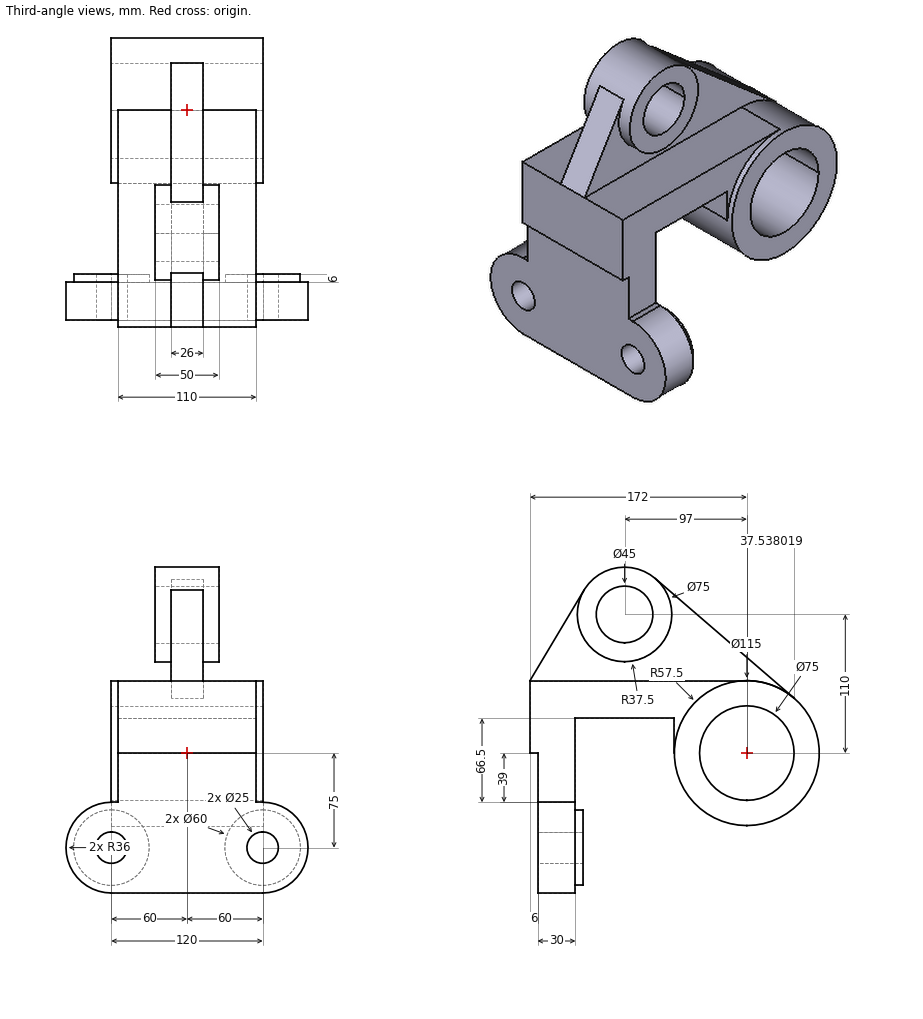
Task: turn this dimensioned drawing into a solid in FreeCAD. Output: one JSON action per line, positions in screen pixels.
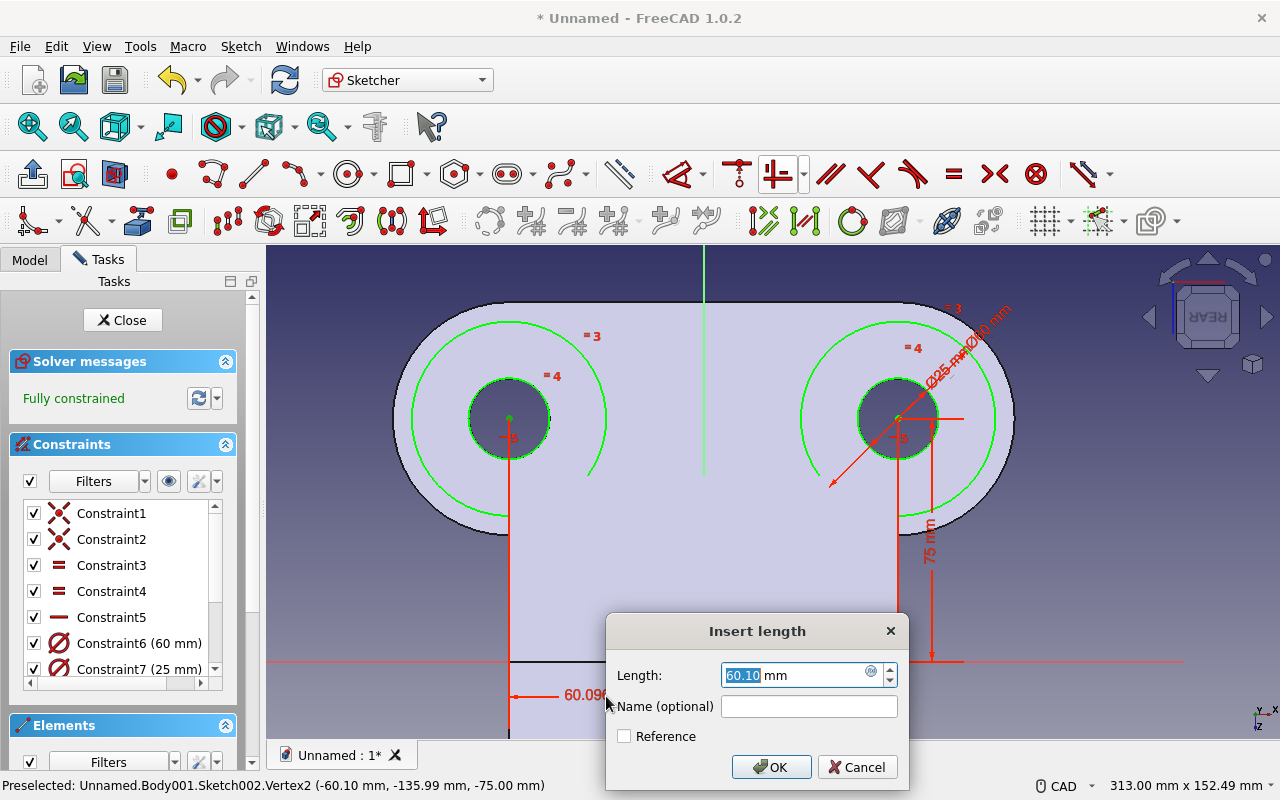
{"action": "type", "text": "60"}
{"action": "key", "text": "Return"}
{"action": "key", "text": "Escape"}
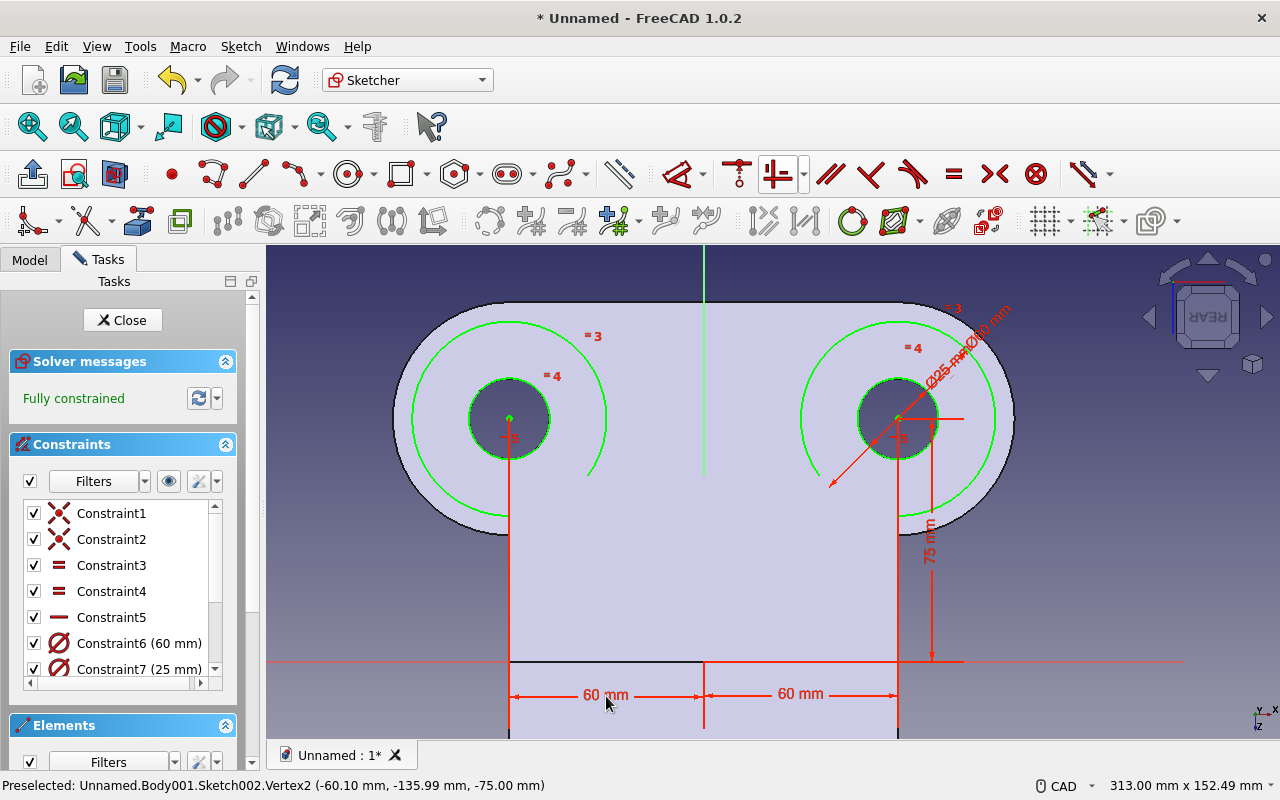
{"action": "left_click", "coordinate": [123, 320]}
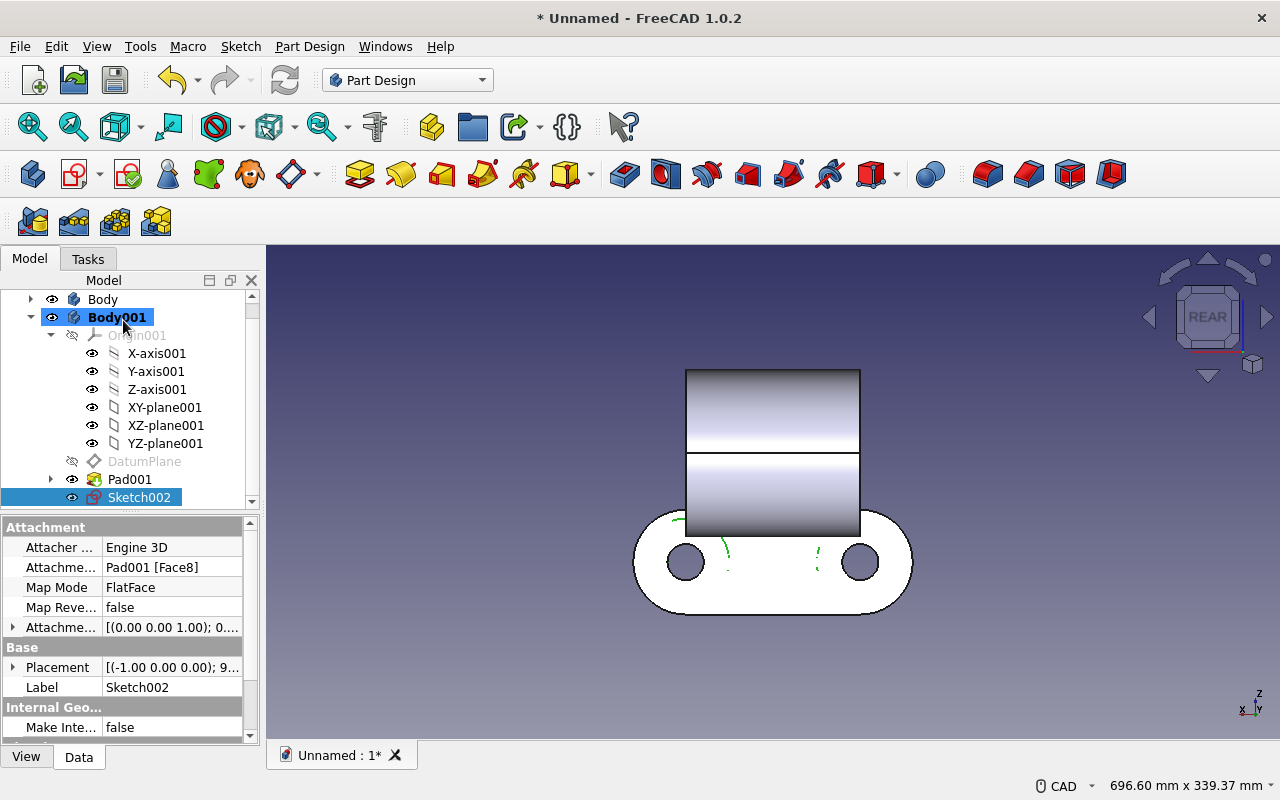
{"action": "left_click", "coordinate": [360, 174]}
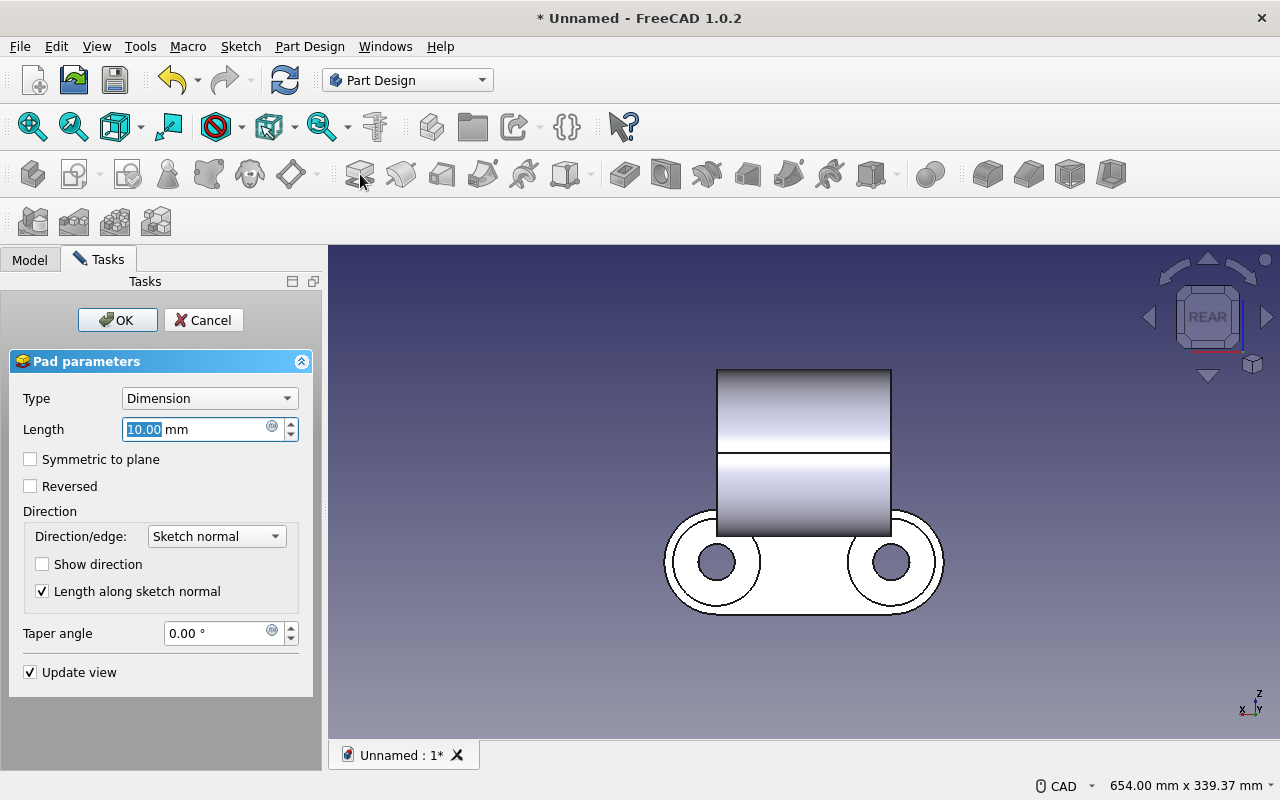
{"action": "type", "text": "6"}
{"action": "key", "text": "Tab"}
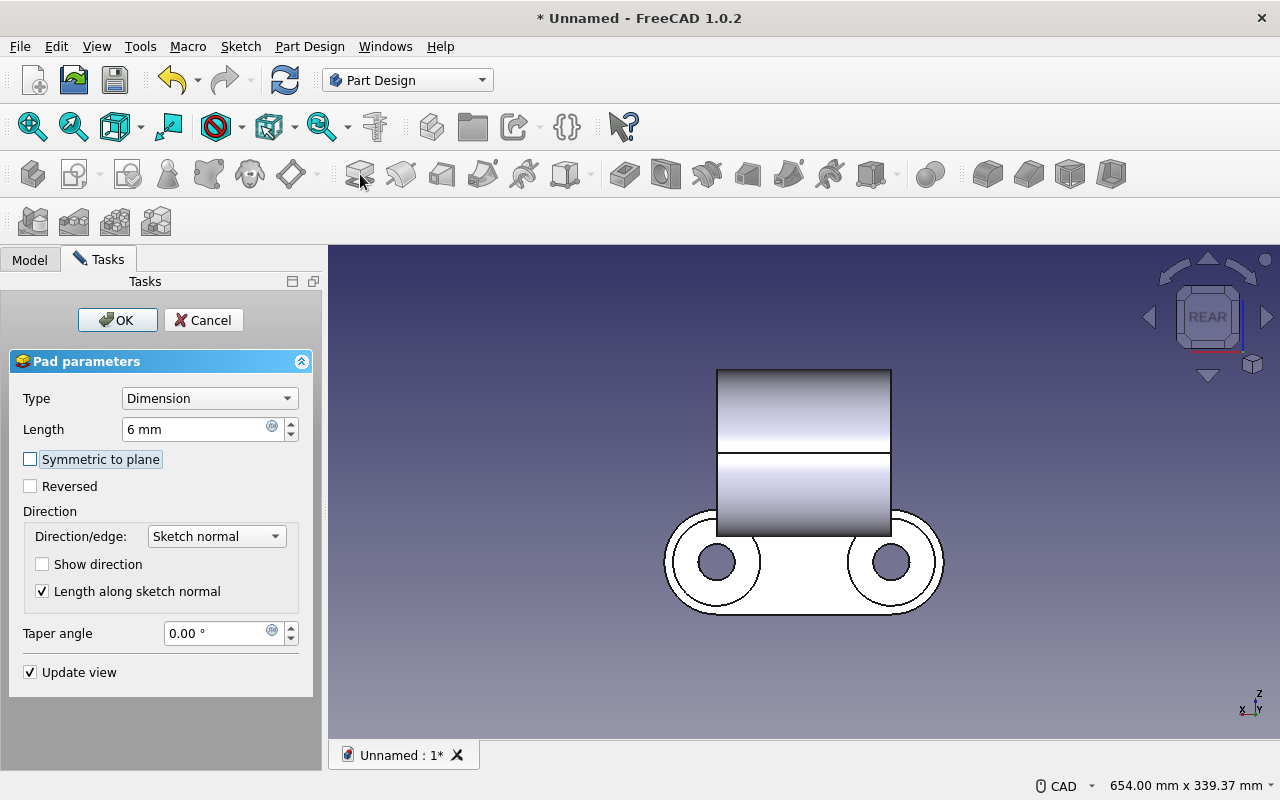
{"action": "left_click", "coordinate": [118, 320]}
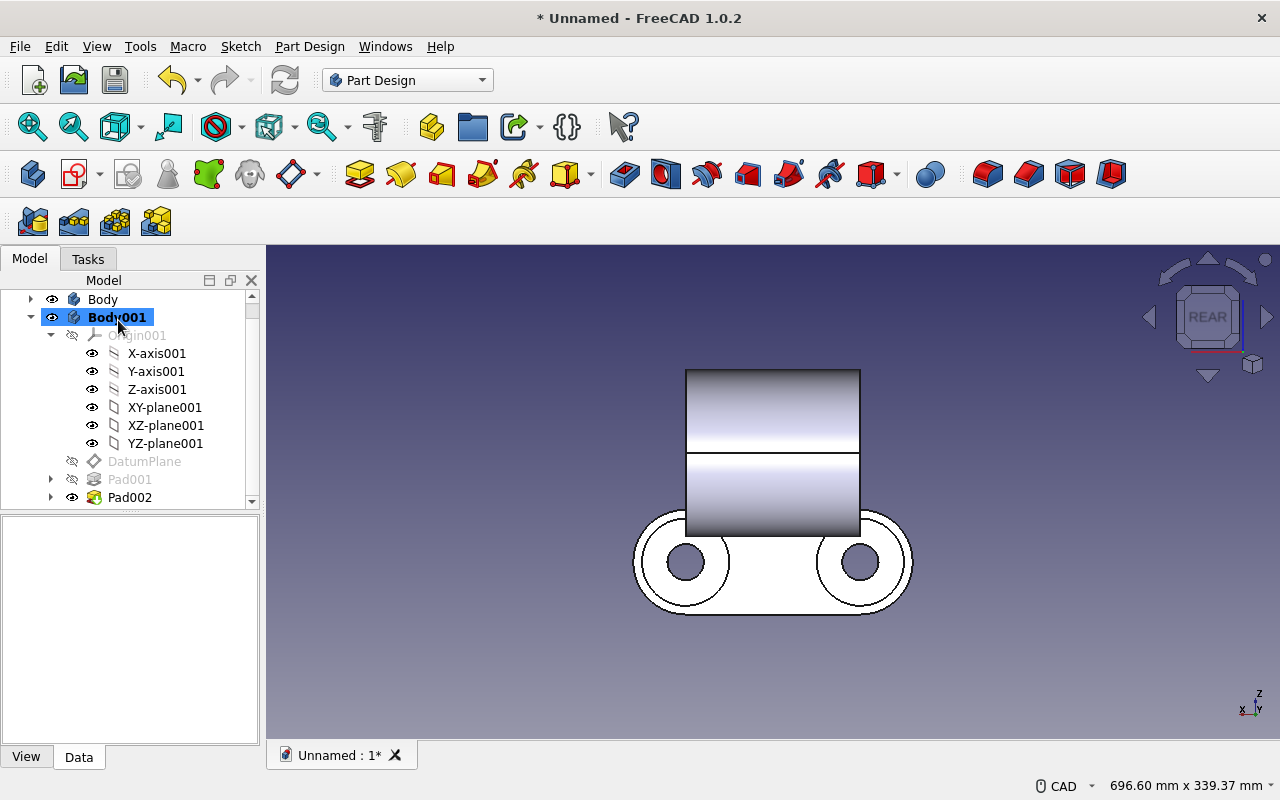
{"action": "key", "text": "v f"}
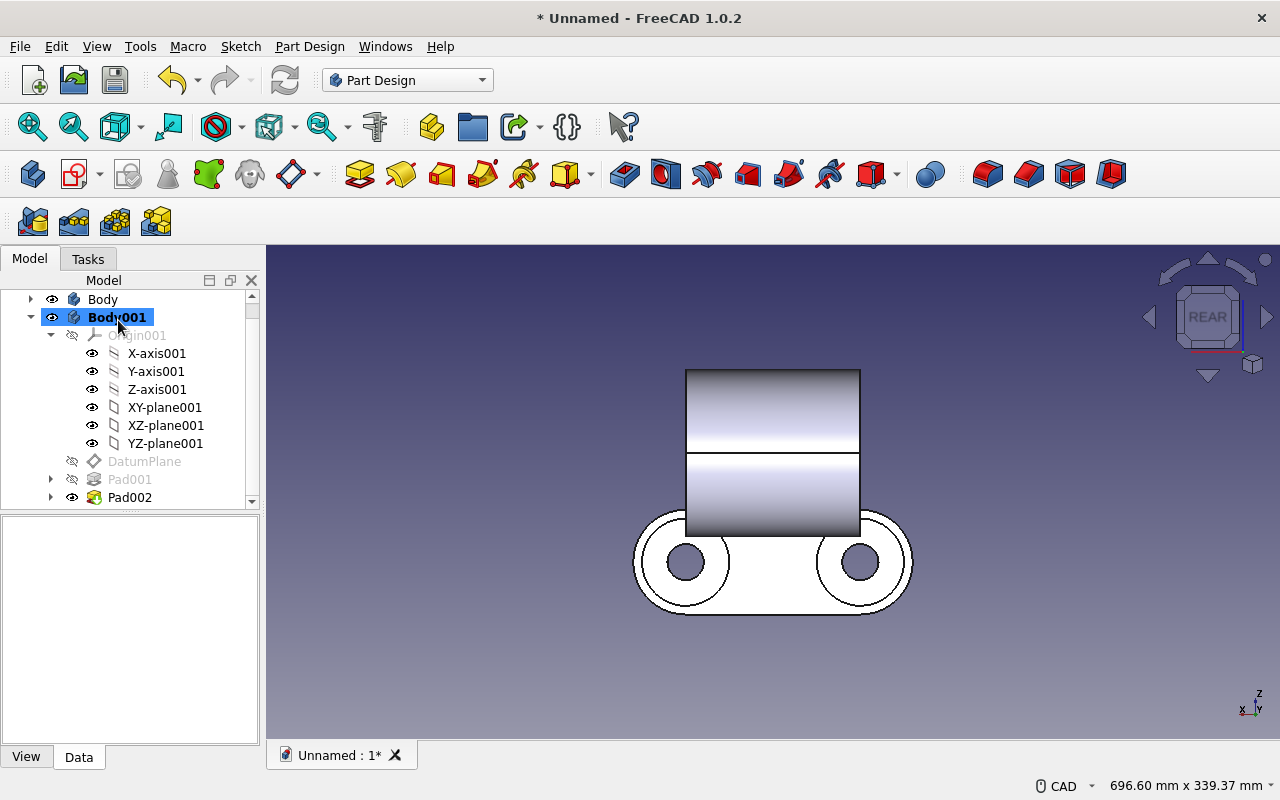
{"action": "double_click", "coordinate": [97, 299]}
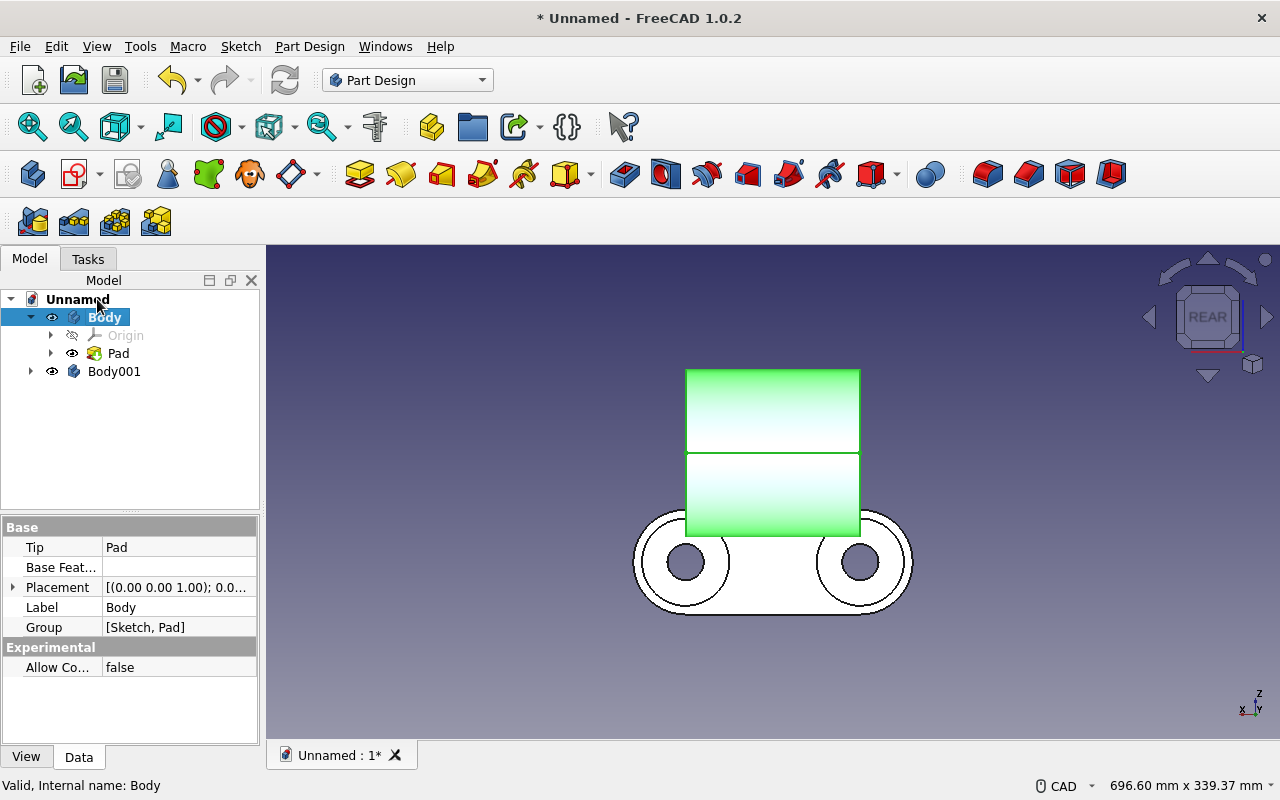
{"action": "left_click", "coordinate": [97, 317]}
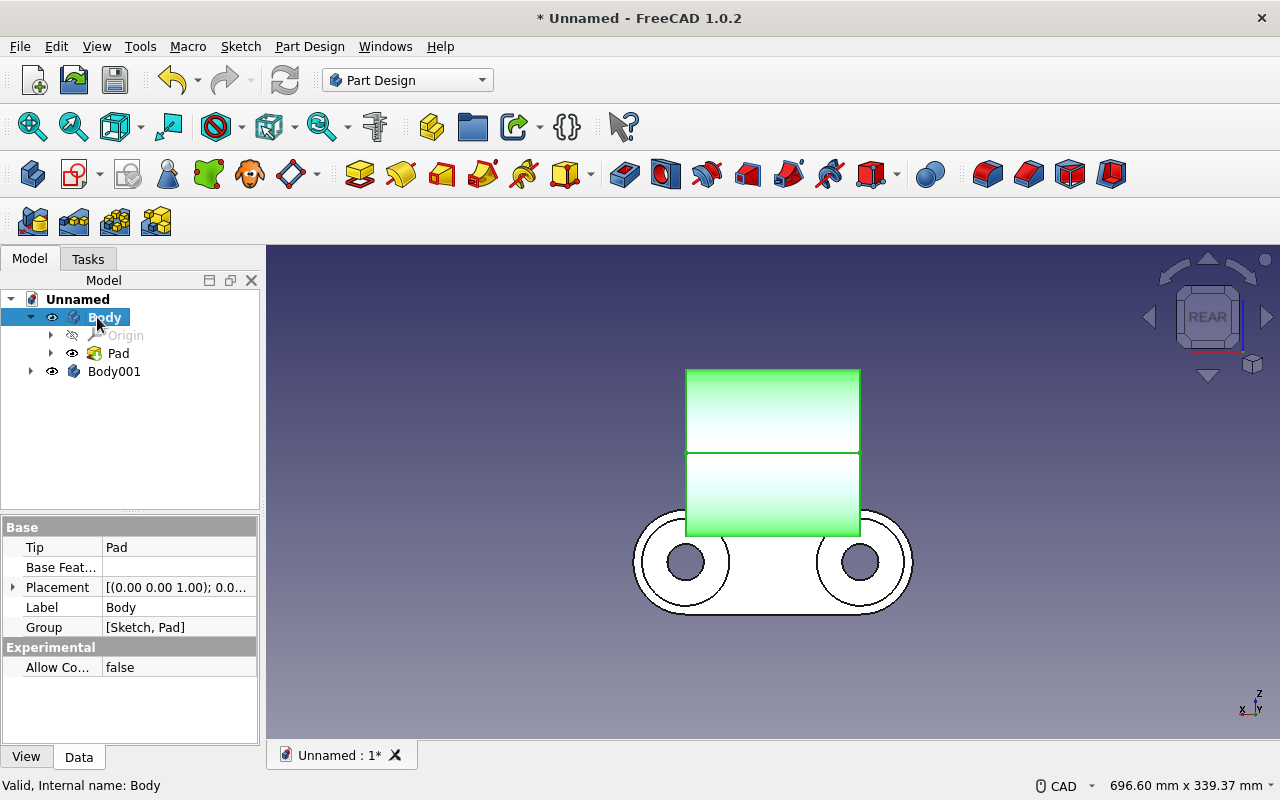
{"action": "left_click", "coordinate": [148, 667]}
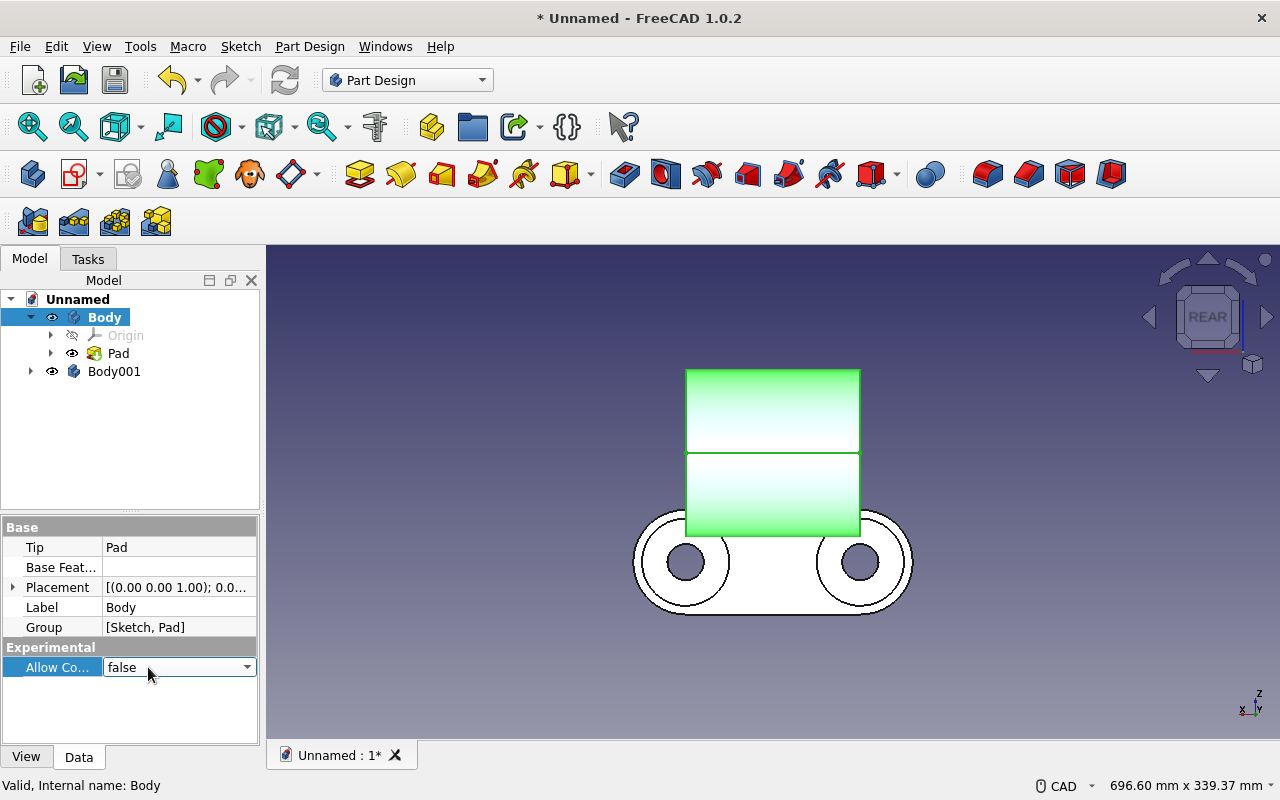
{"action": "left_click", "coordinate": [148, 667]}